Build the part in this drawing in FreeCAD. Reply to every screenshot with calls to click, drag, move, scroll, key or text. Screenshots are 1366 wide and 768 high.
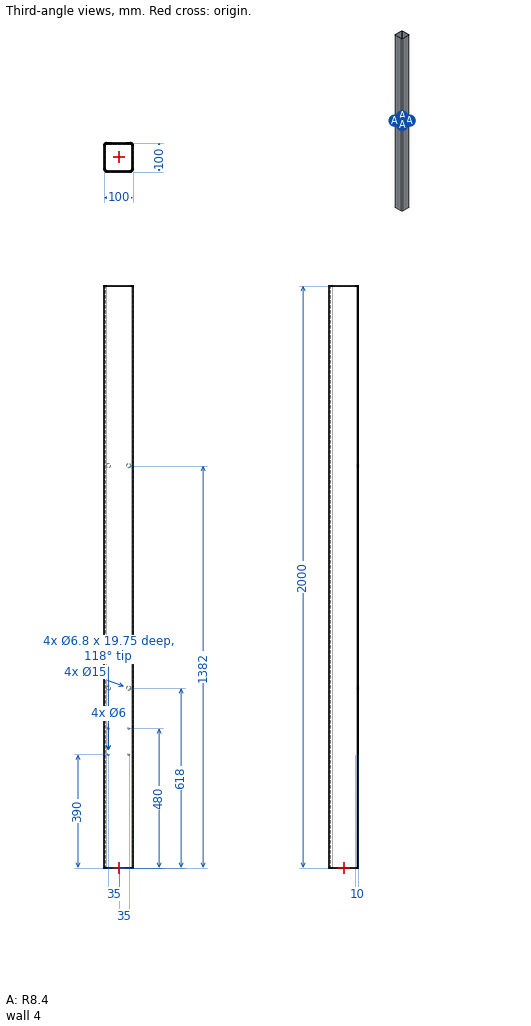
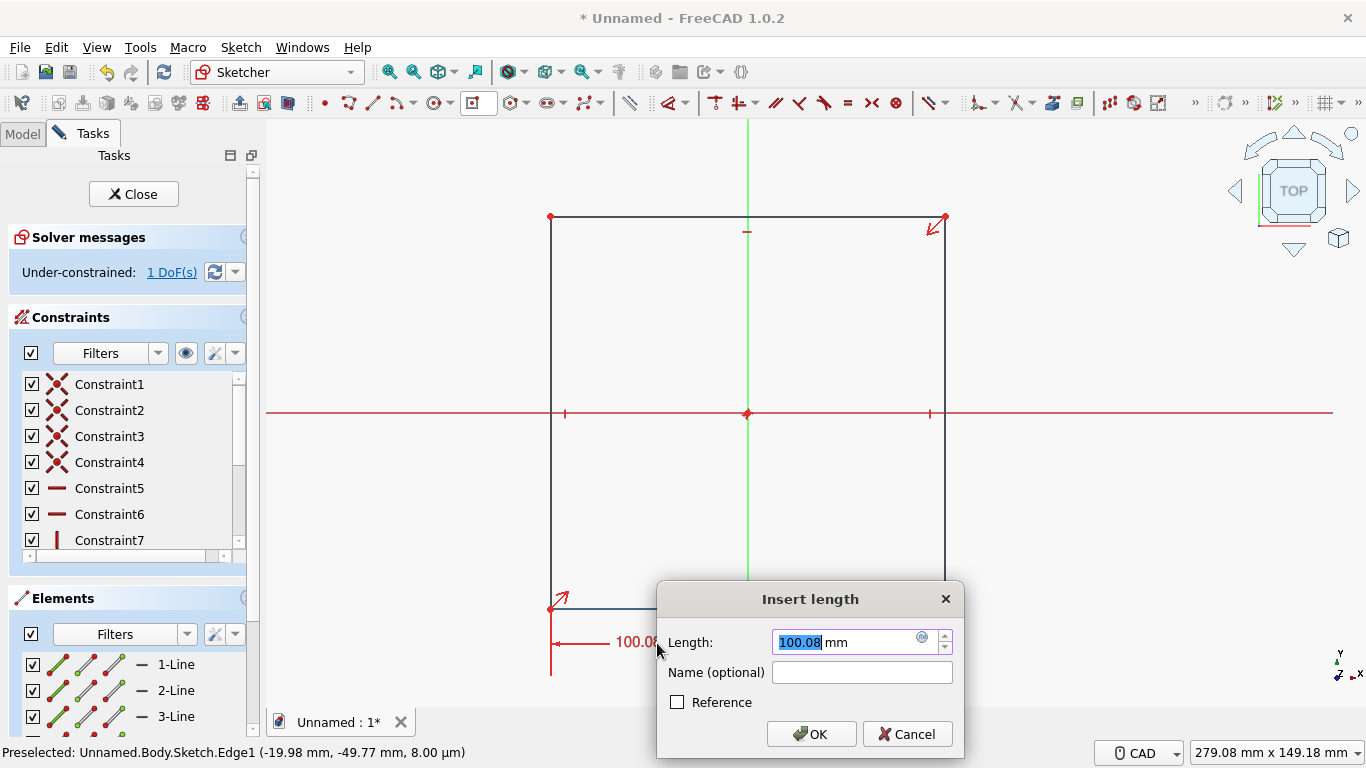
text(100)
key(Return)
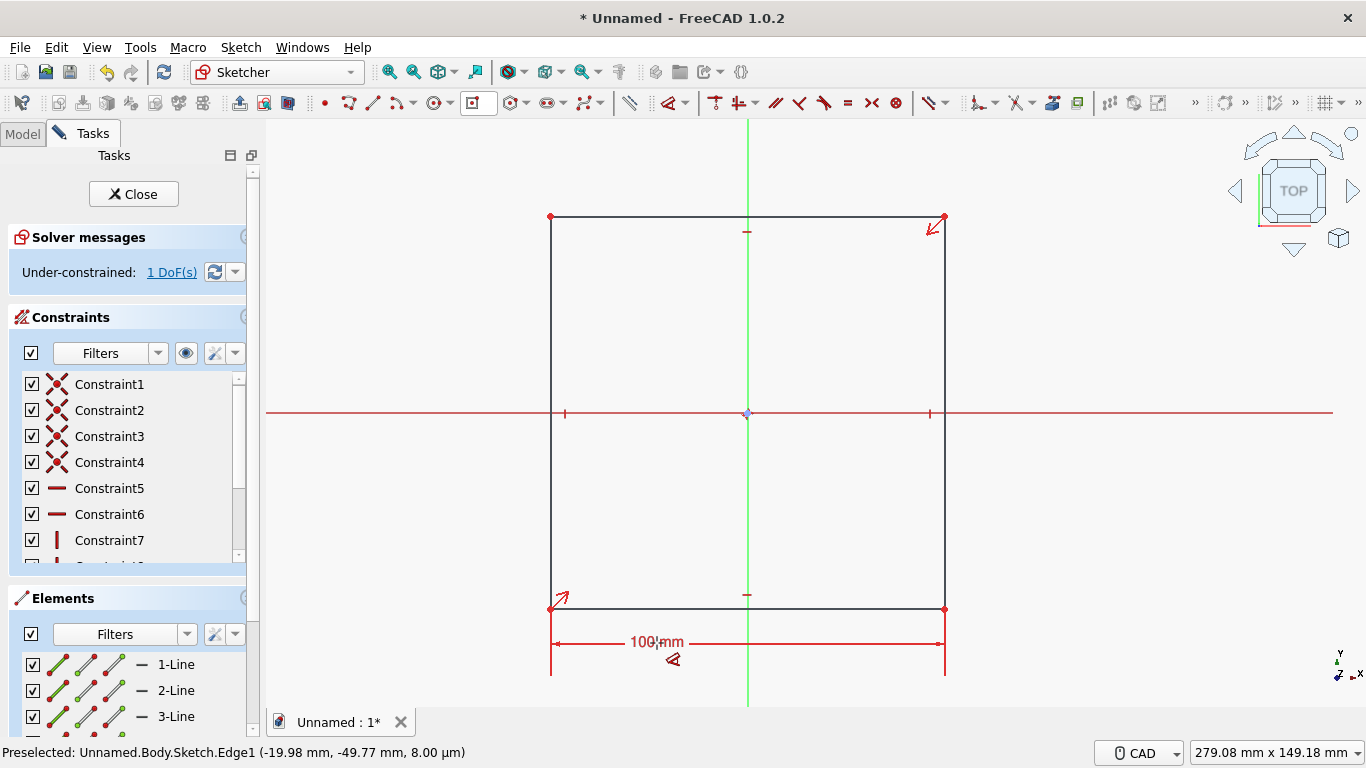
click(945, 492)
click(979, 323)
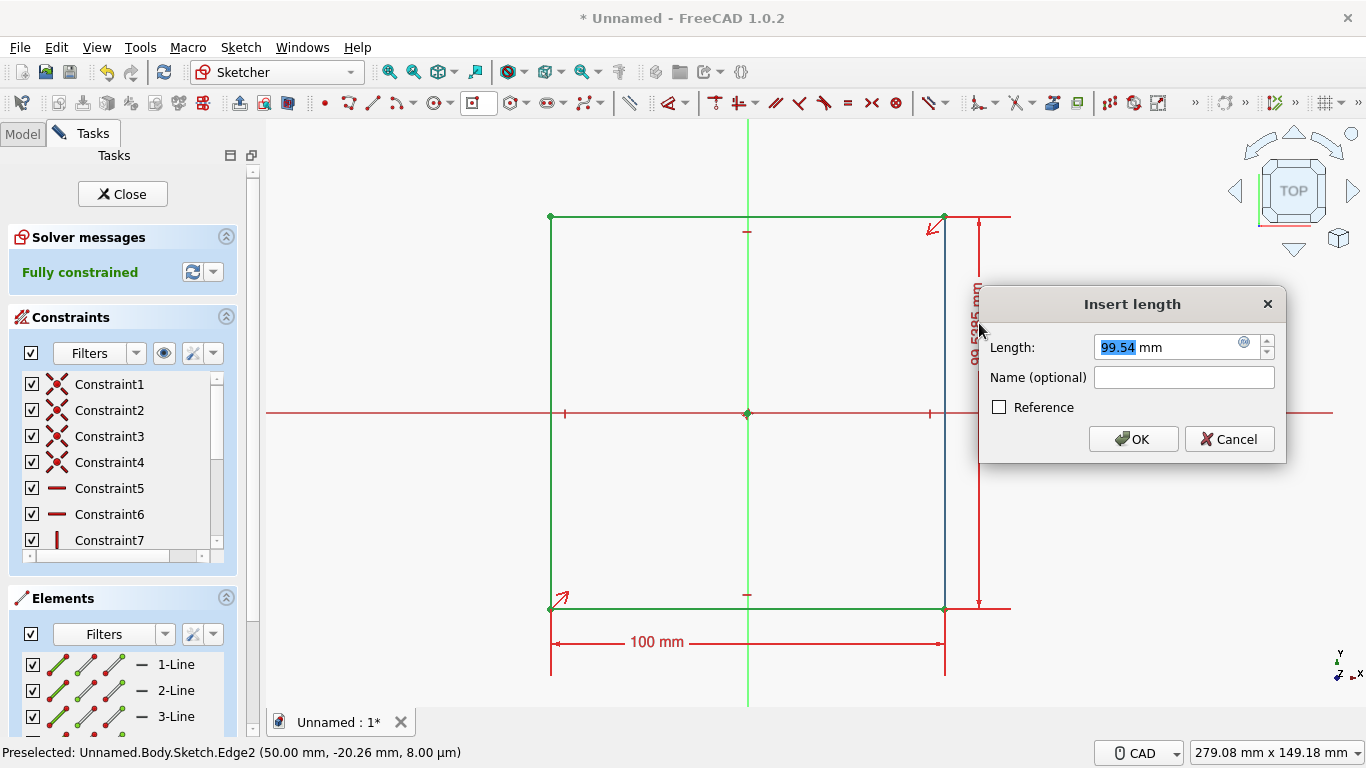
text(100)
key(Return)
key(Escape)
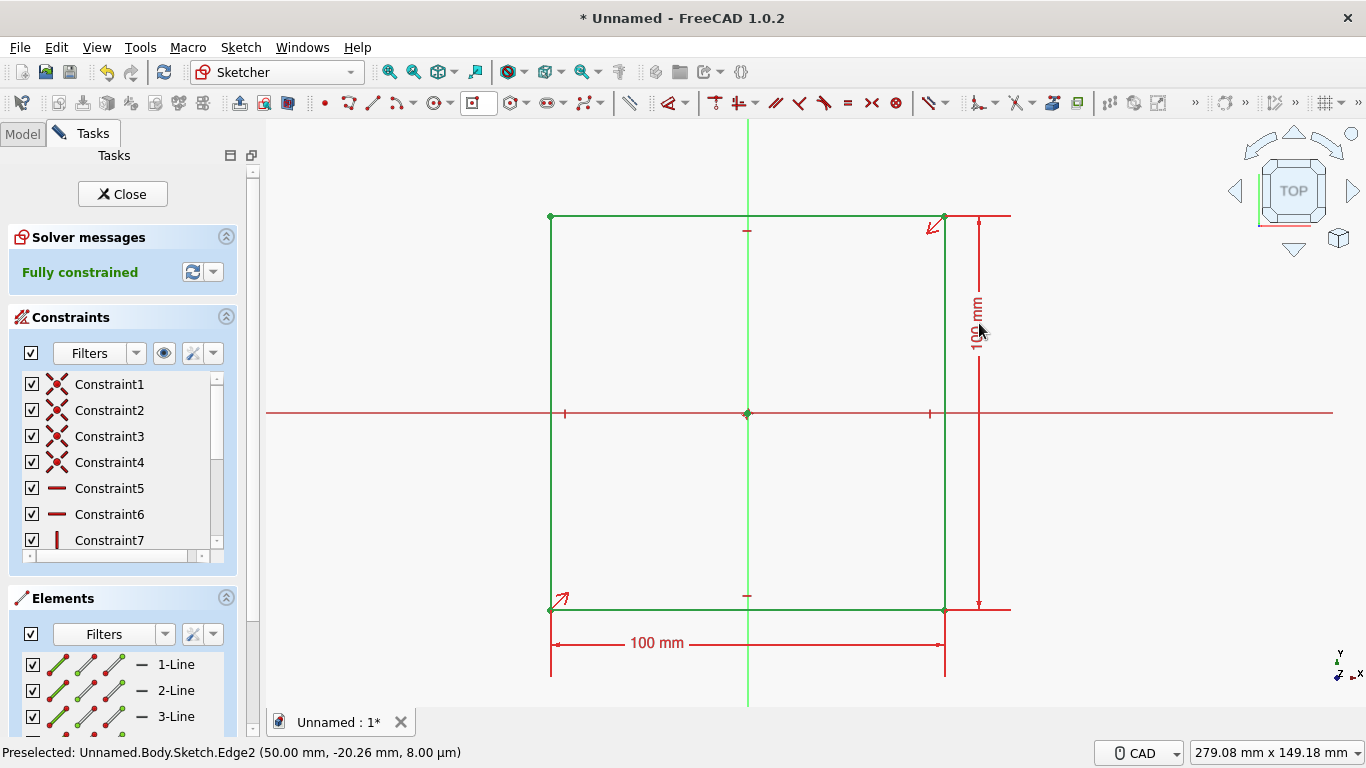
click(123, 194)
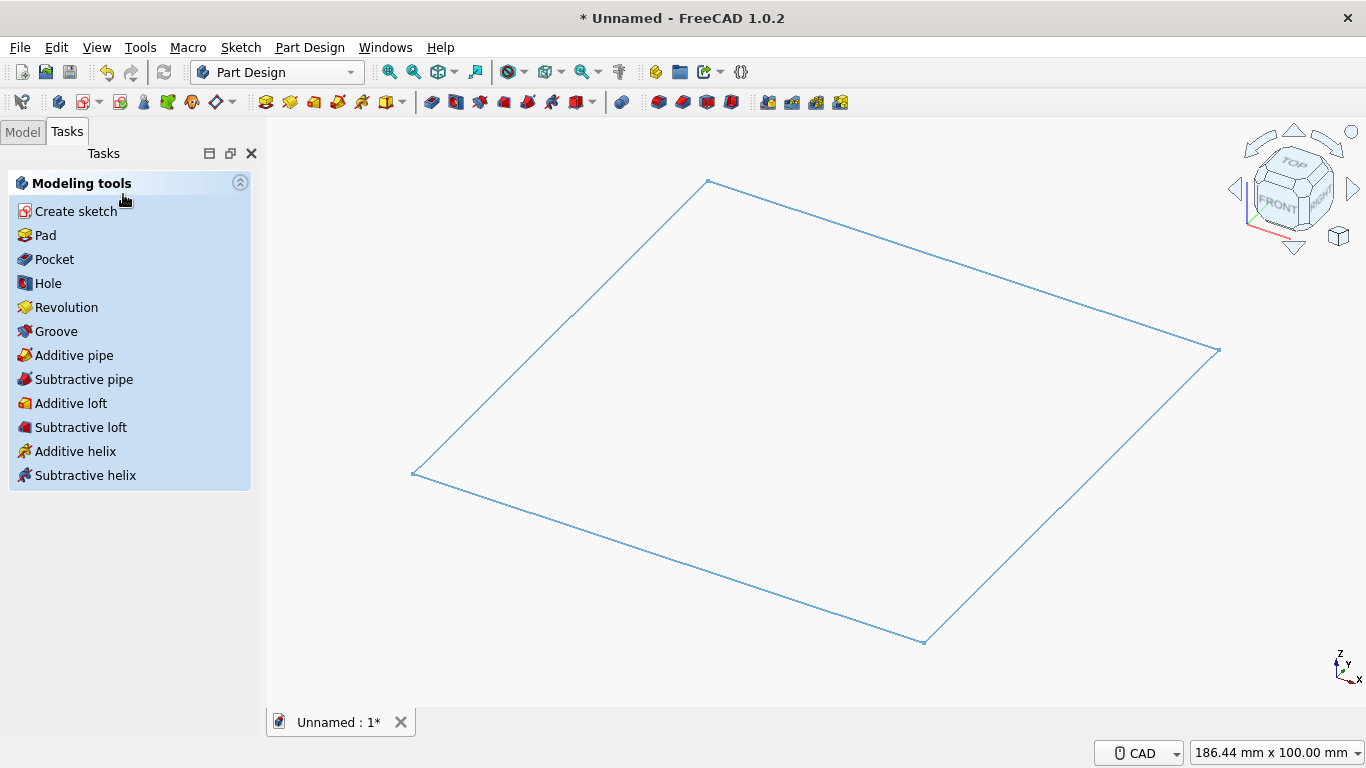
click(266, 102)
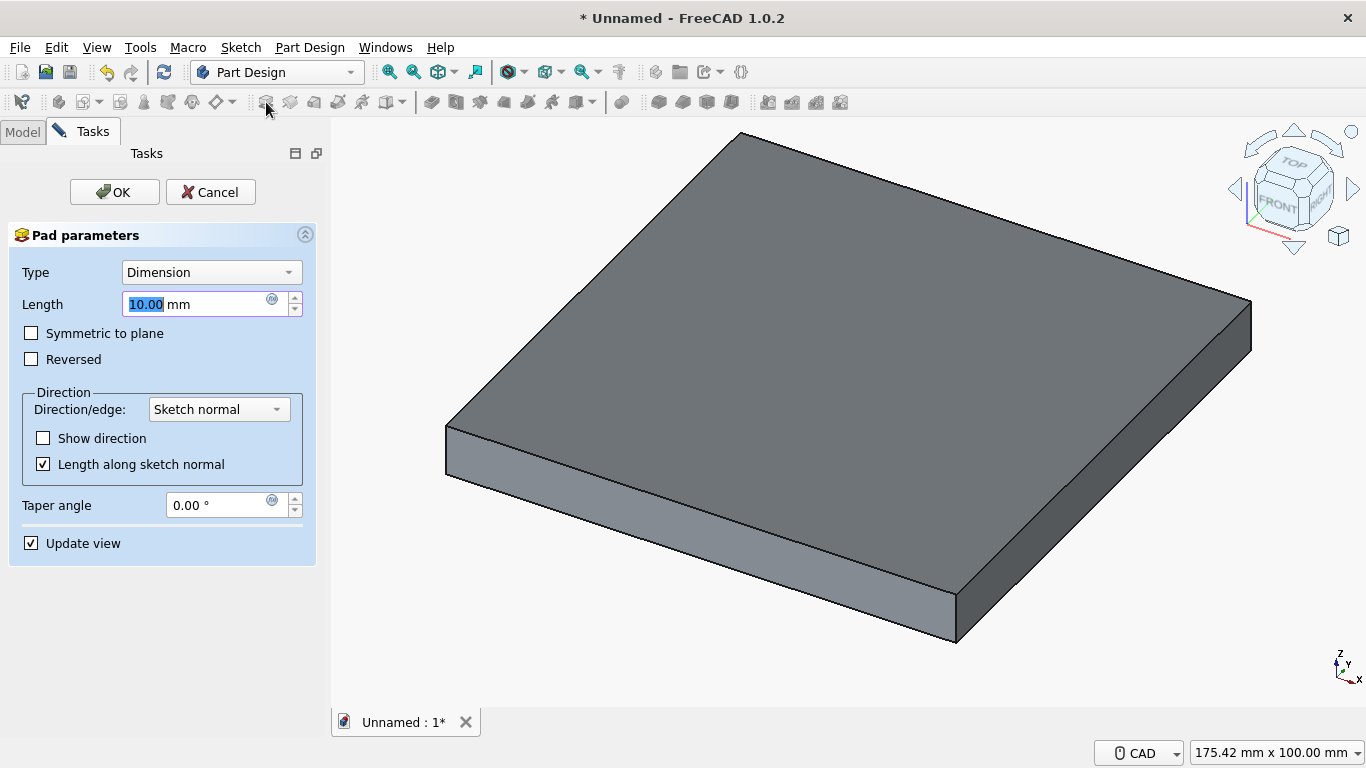
text(2000)
key(Tab)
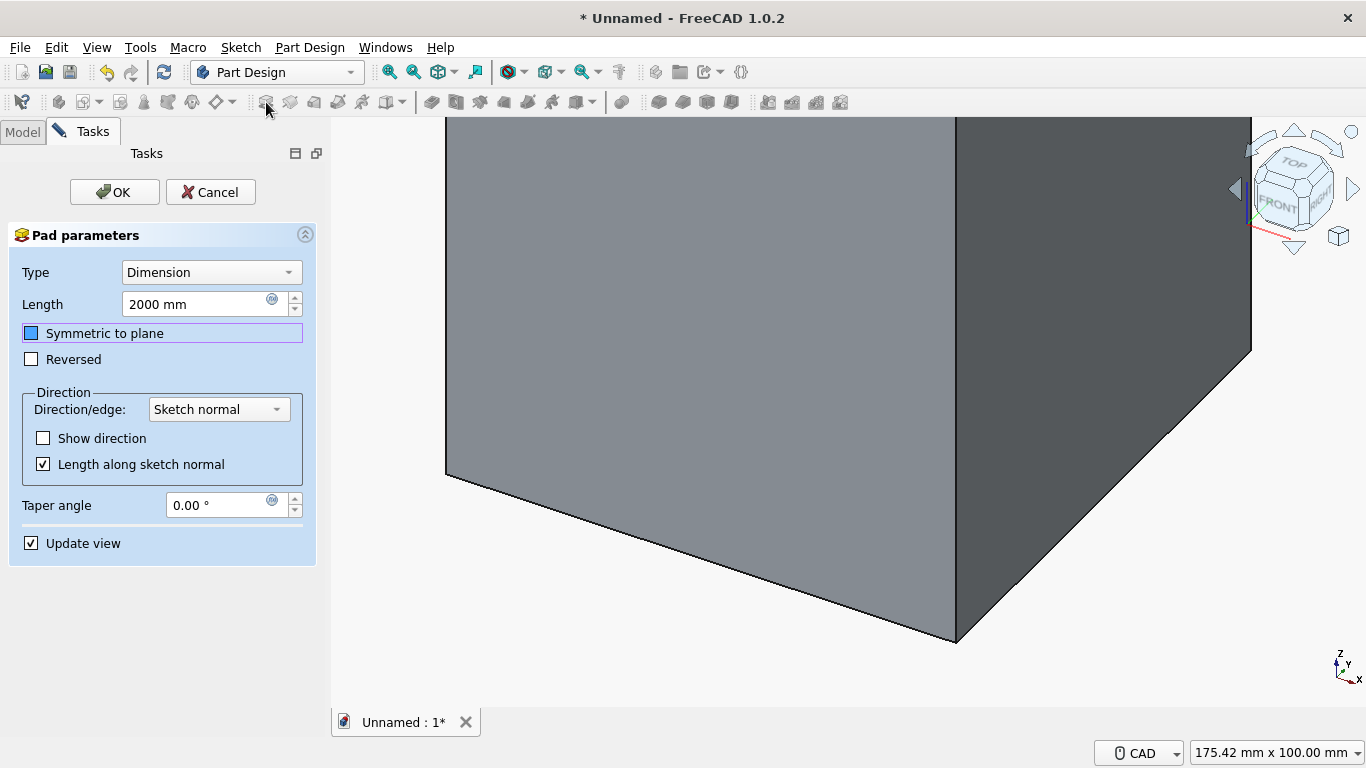
click(115, 192)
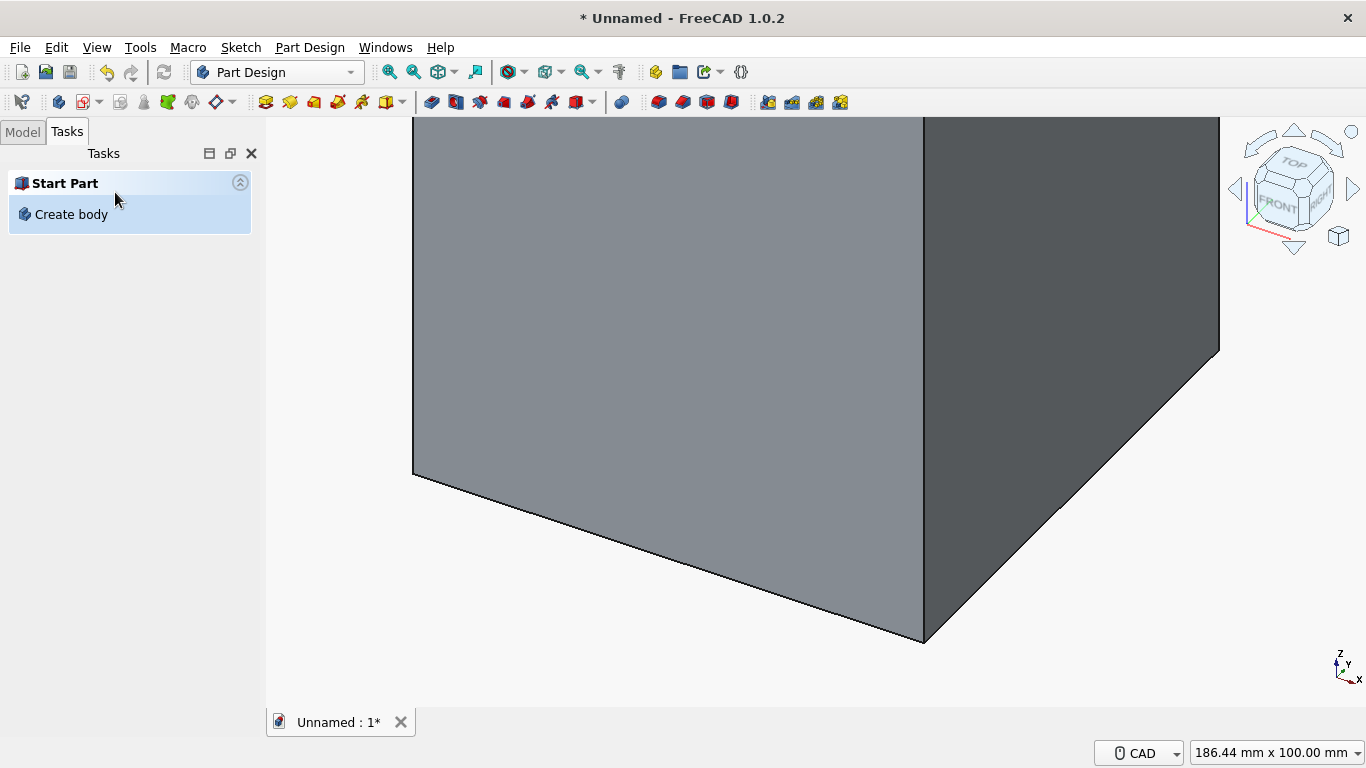
click(390, 72)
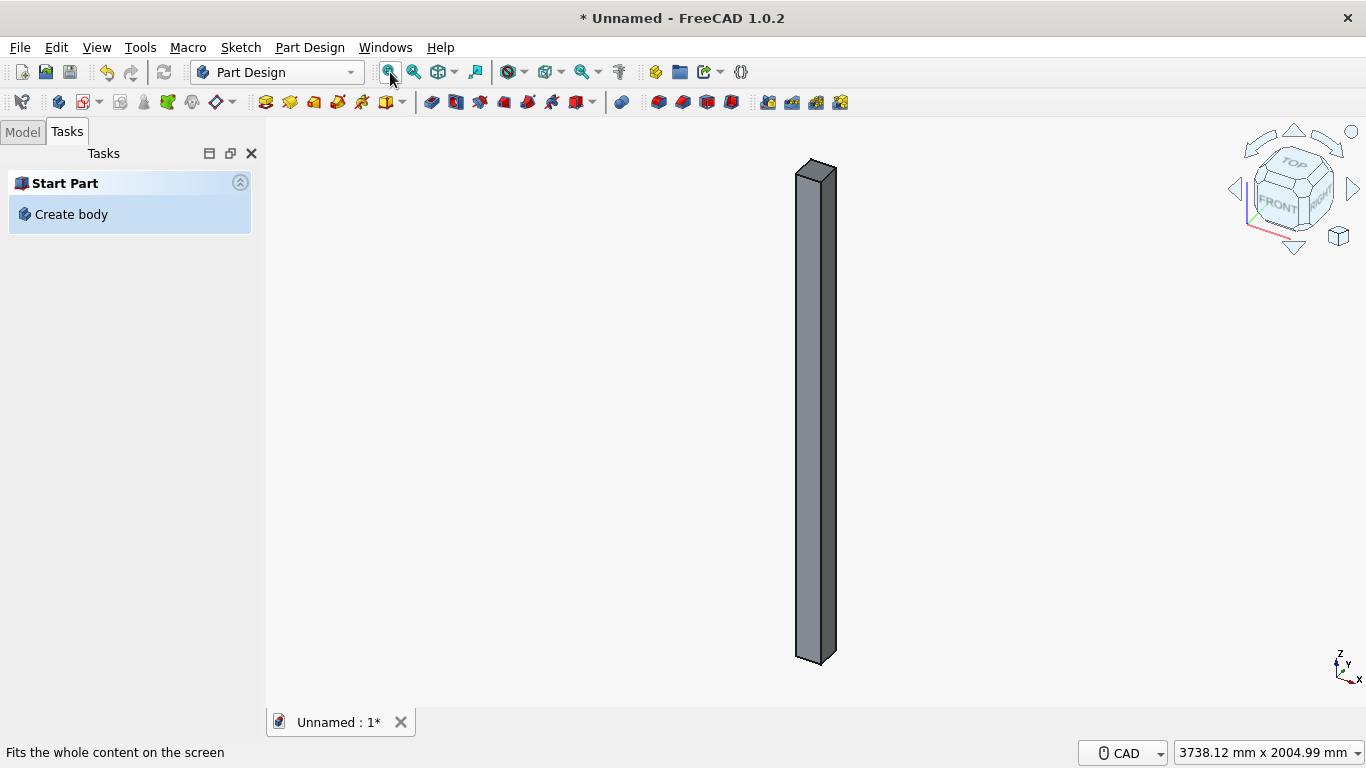
click(821, 423)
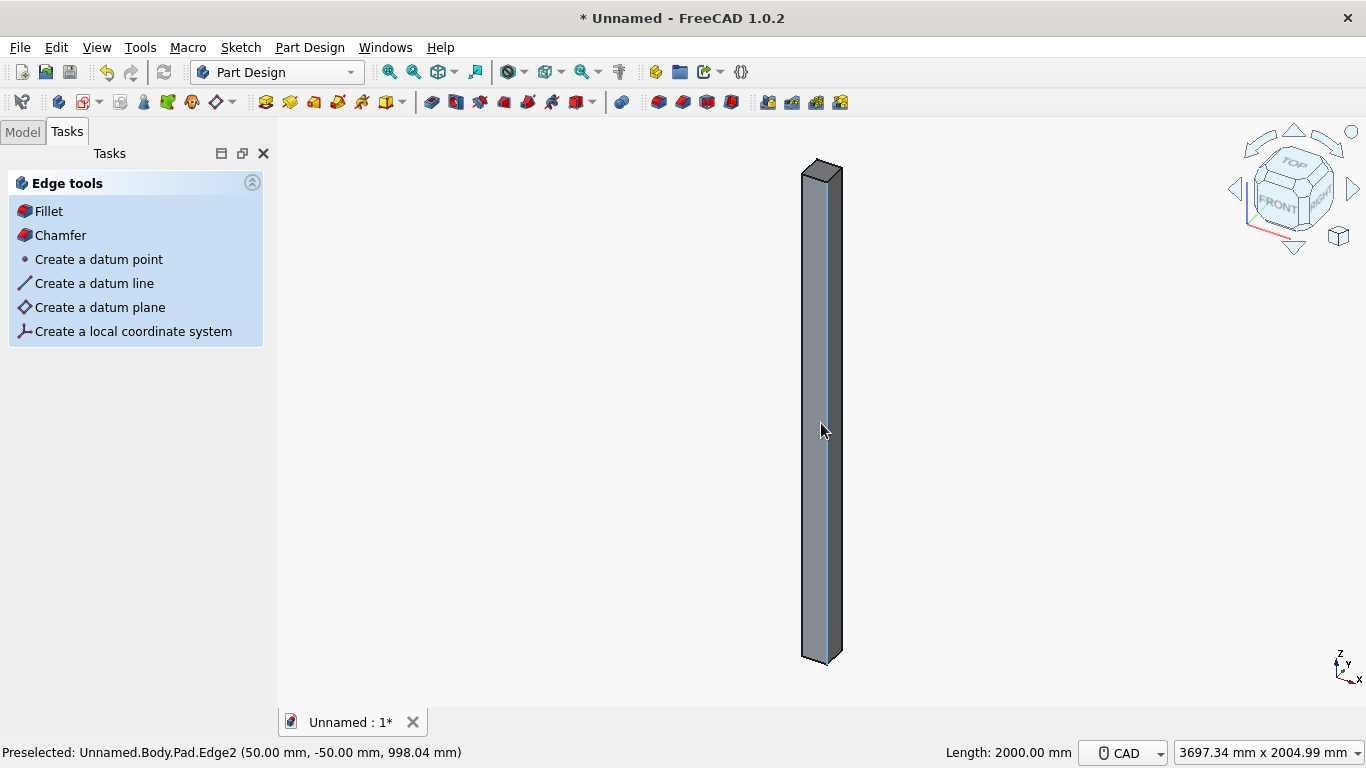
key(0)